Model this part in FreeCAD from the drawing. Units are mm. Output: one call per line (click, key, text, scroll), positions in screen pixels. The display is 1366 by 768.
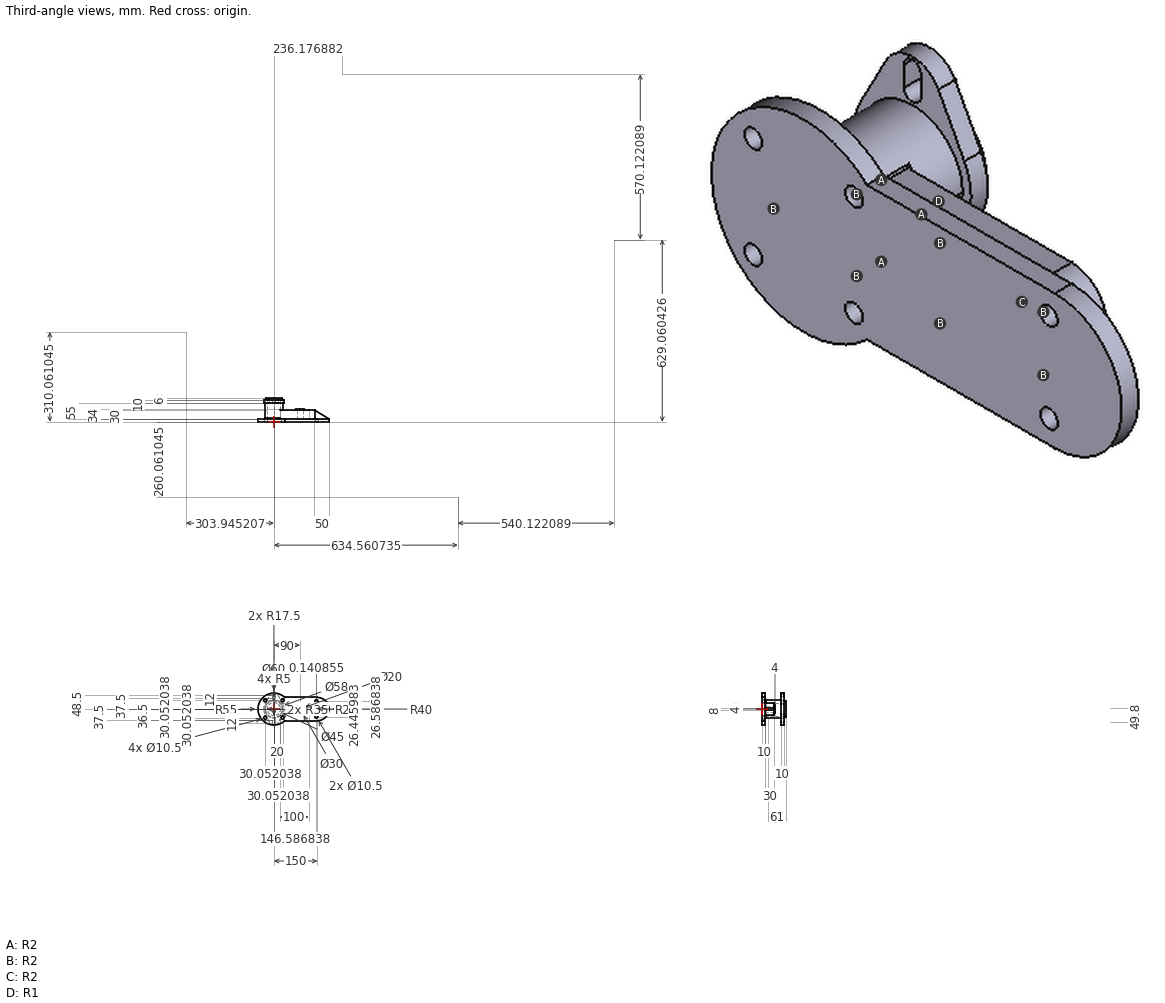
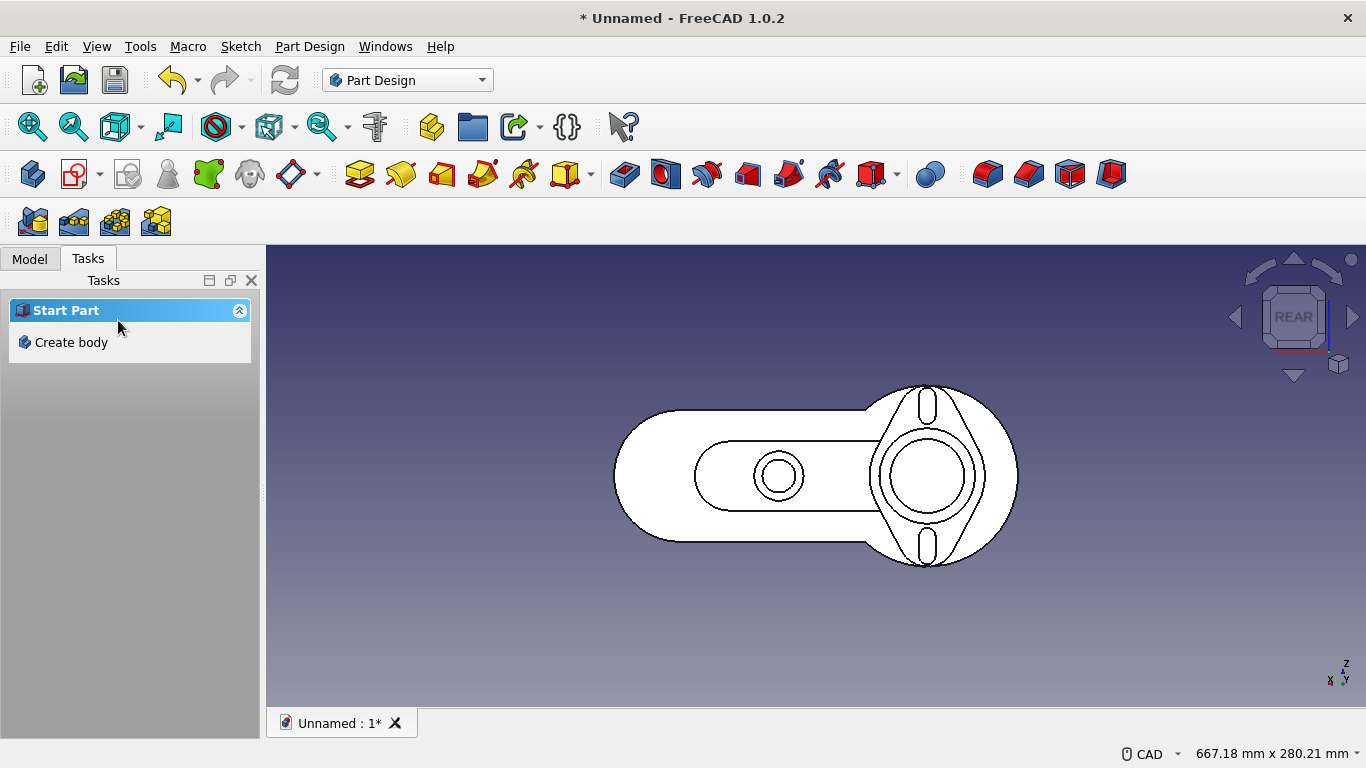
key(v)
key(f)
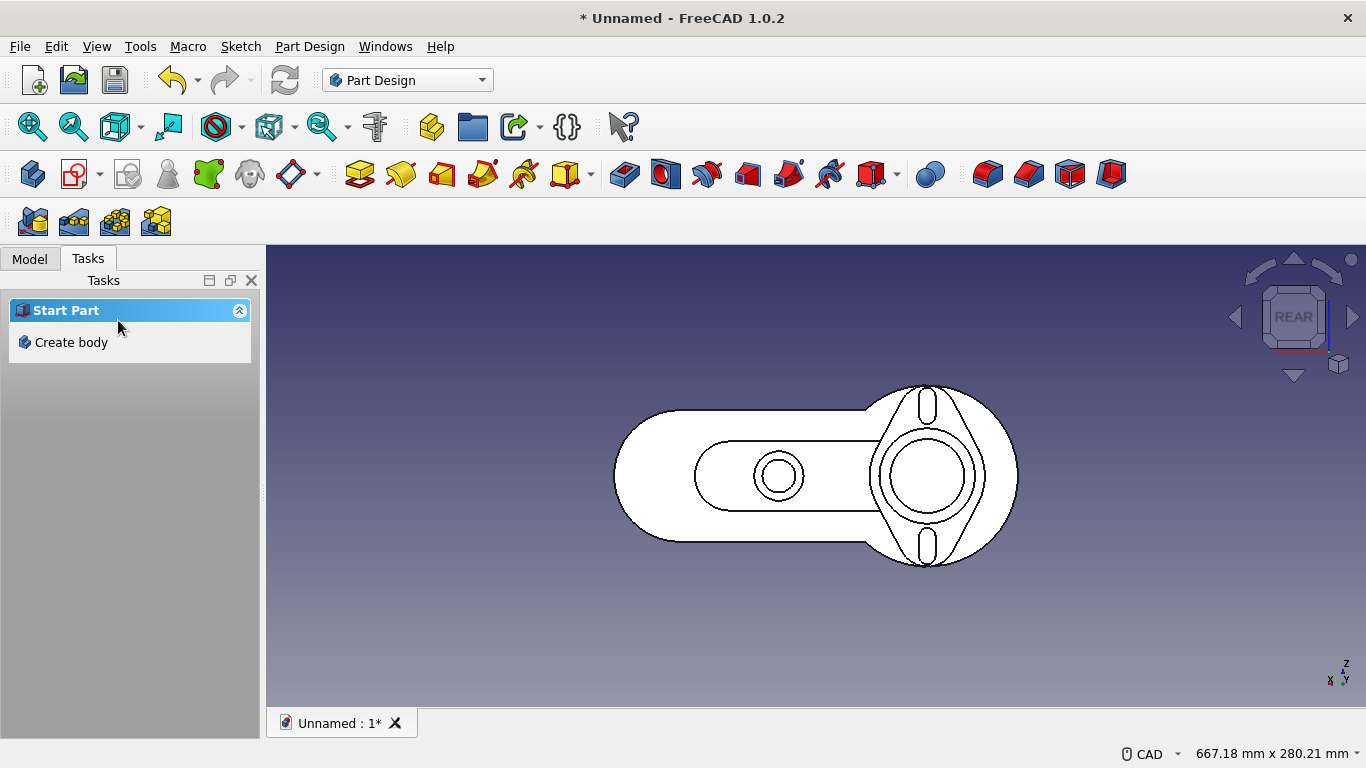
click(643, 475)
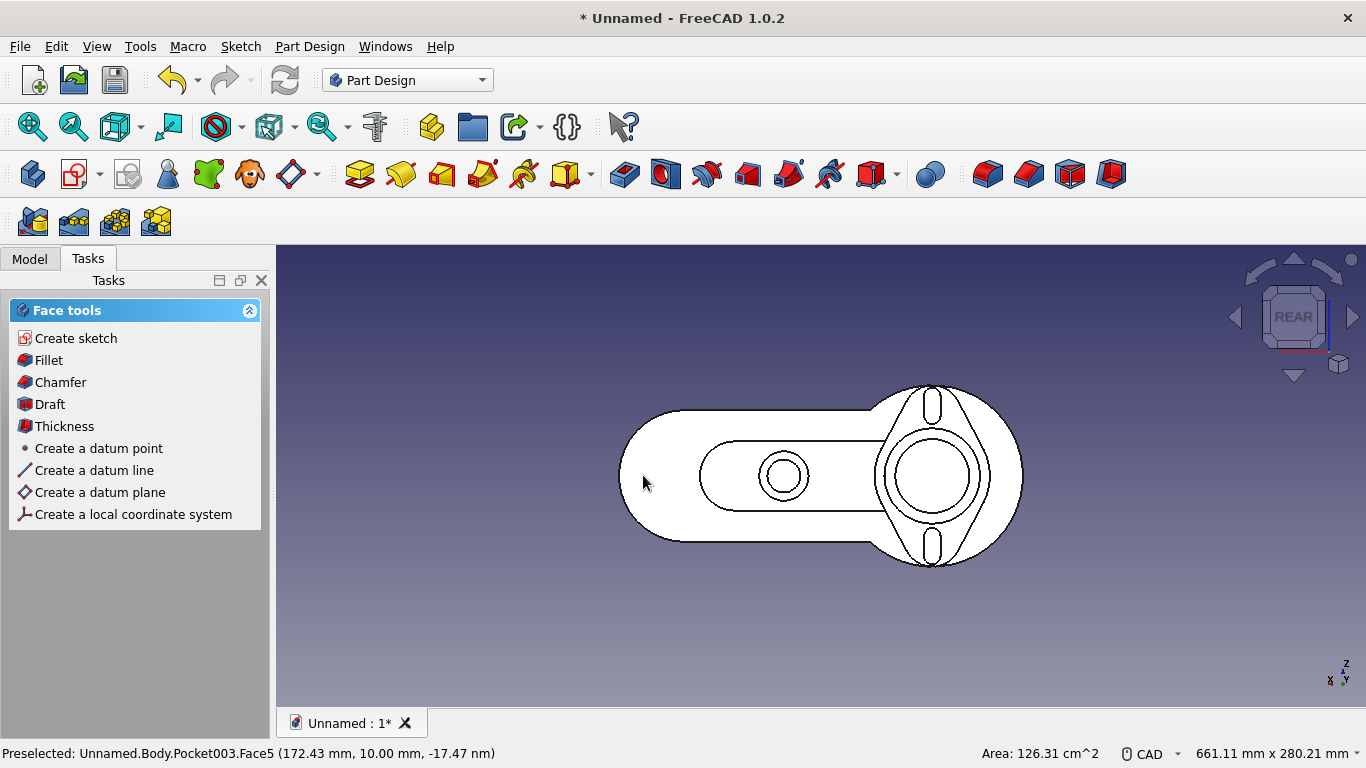
click(74, 174)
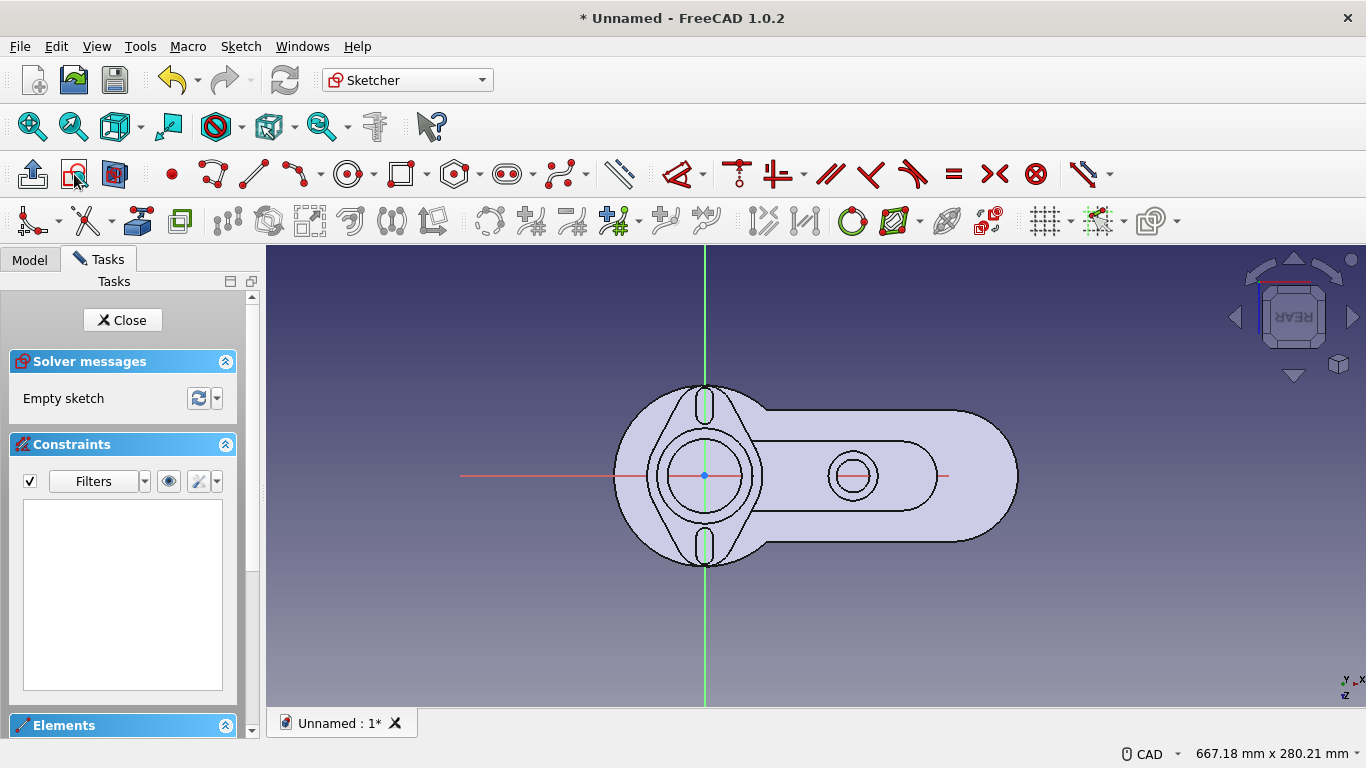
click(115, 174)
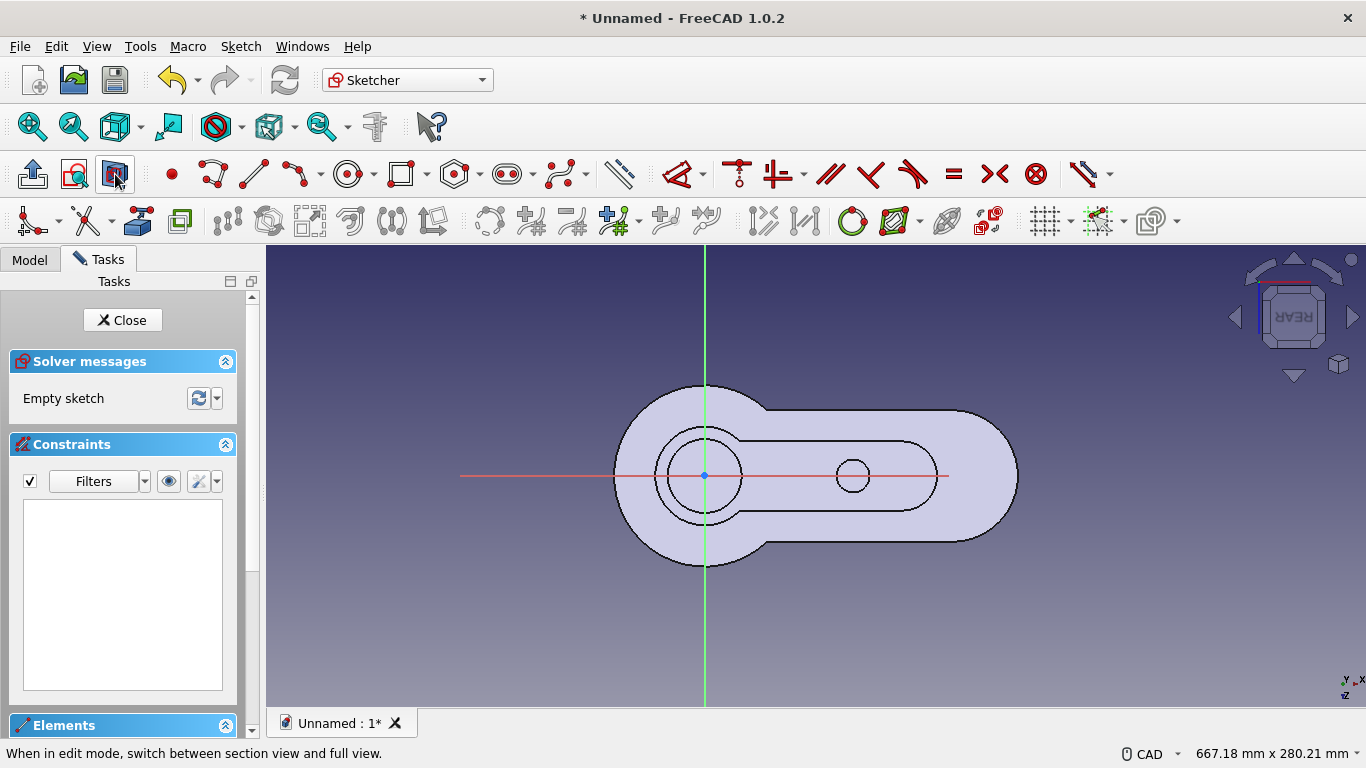
scroll(680, 476, up, 5)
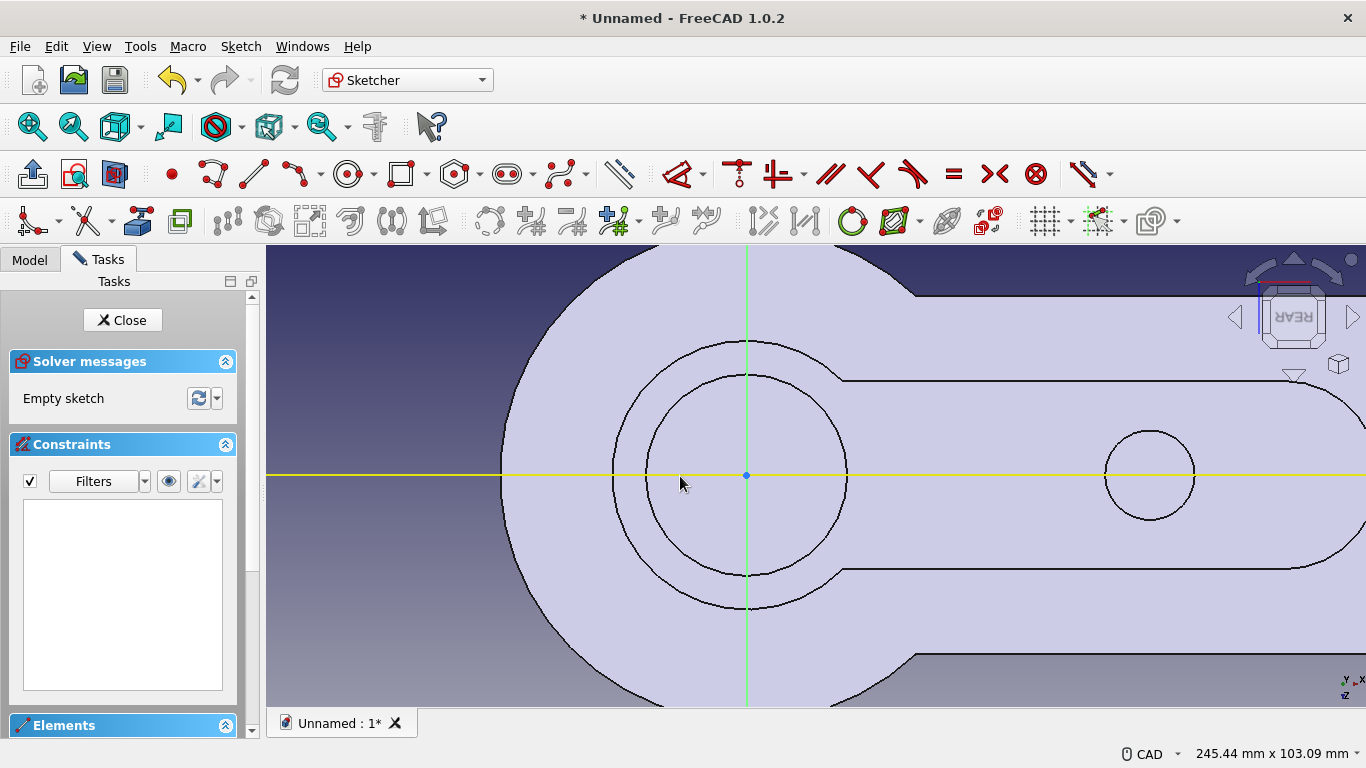
key(g)
key(c)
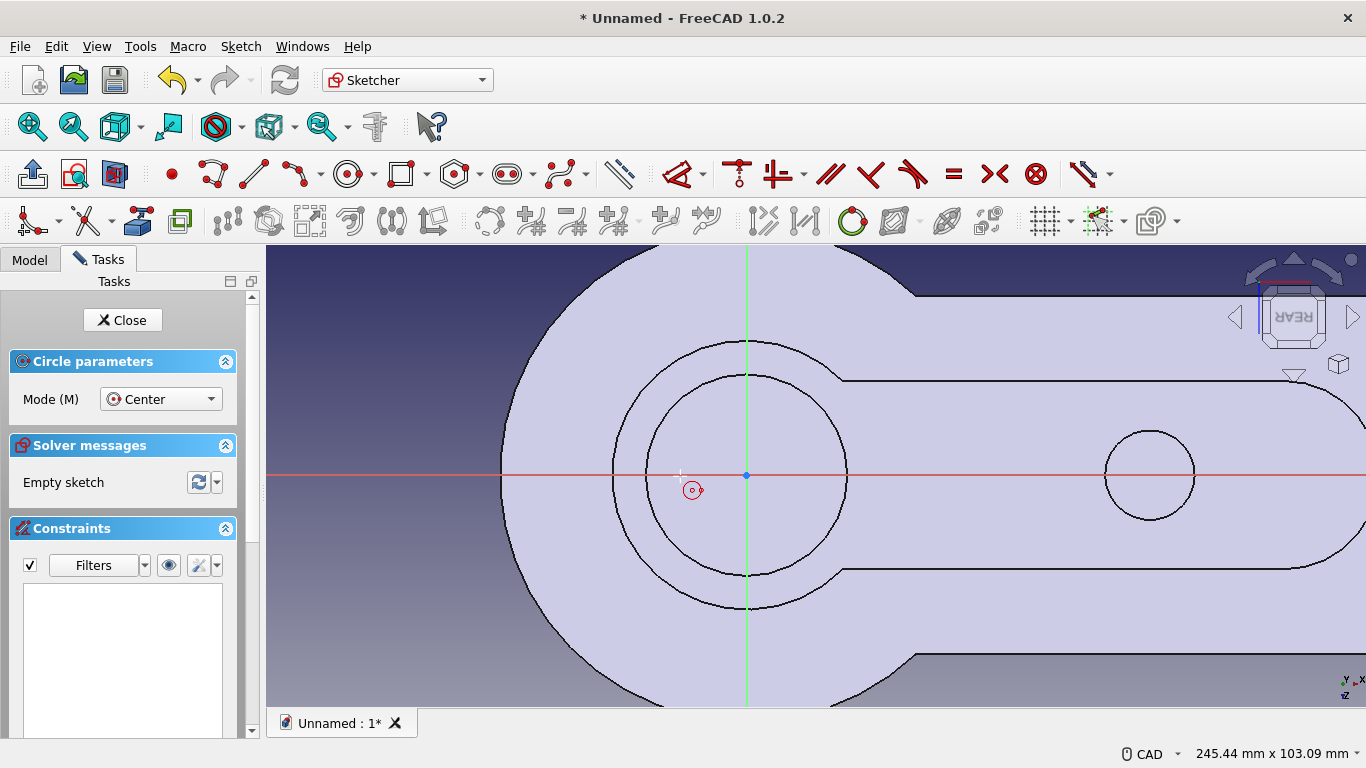
click(612, 340)
click(628, 324)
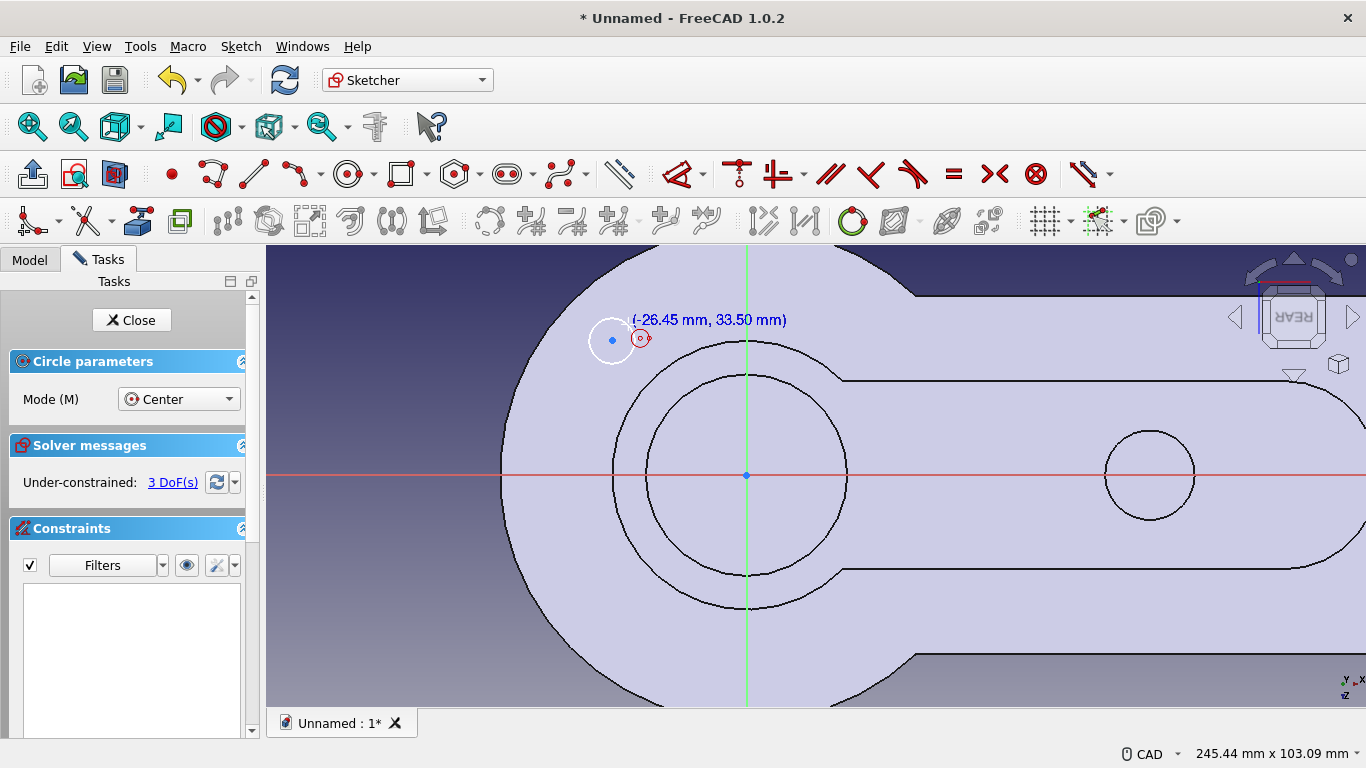
click(881, 340)
click(898, 324)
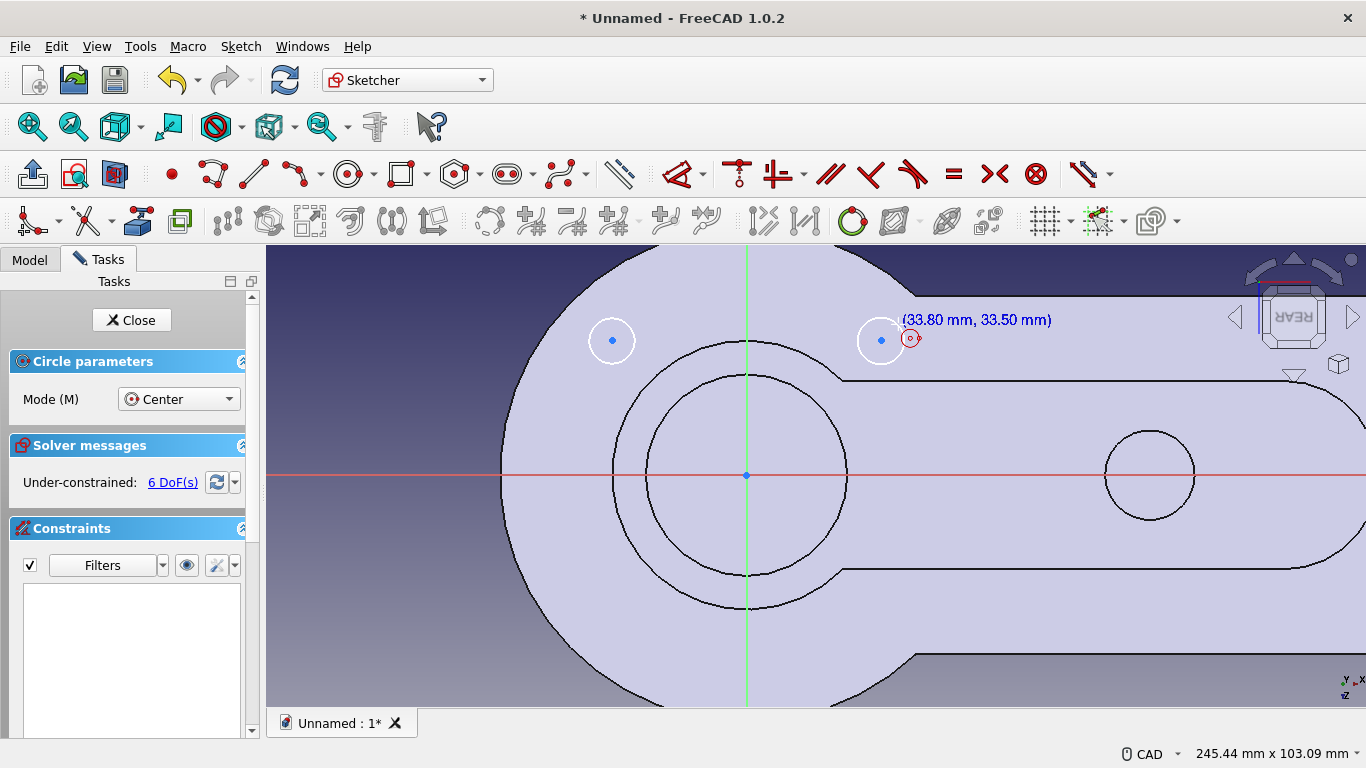
click(881, 610)
click(898, 593)